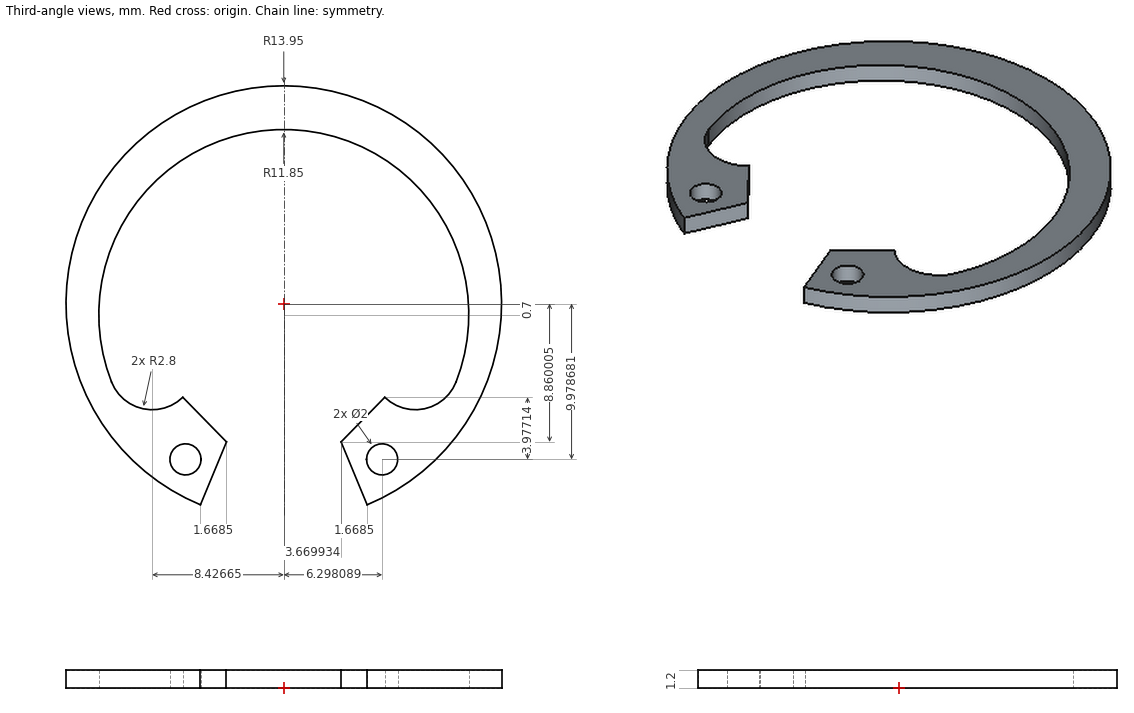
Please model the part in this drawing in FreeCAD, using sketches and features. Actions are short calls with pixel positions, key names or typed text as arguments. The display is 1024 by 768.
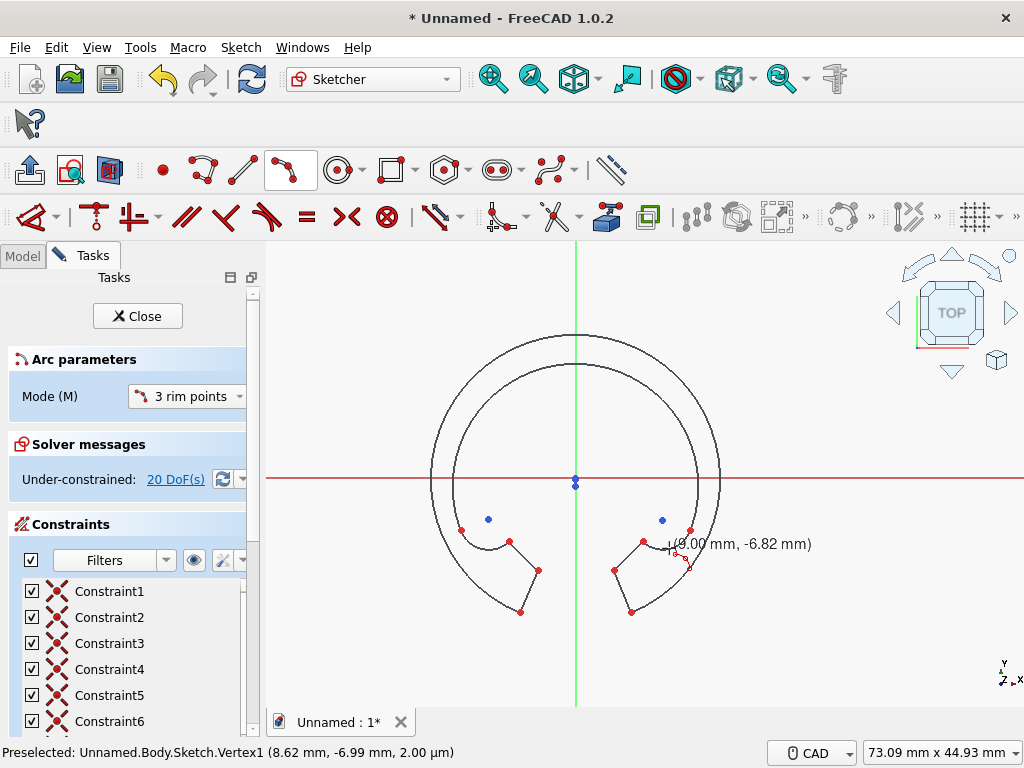
click(338, 170)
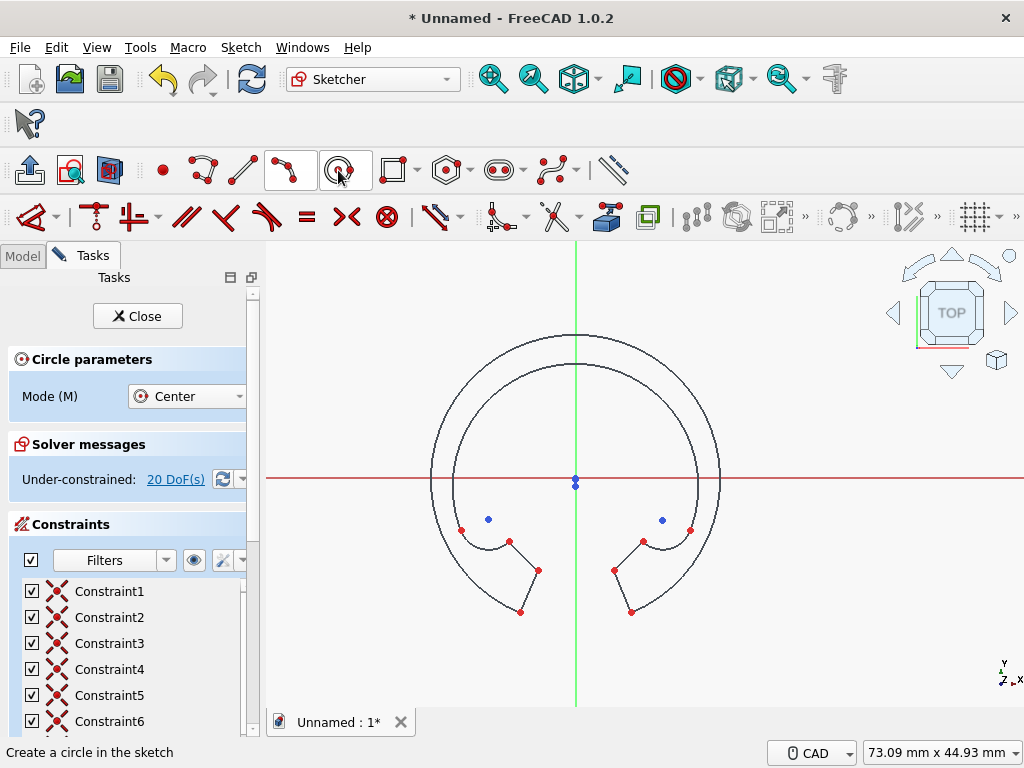
scroll(641, 582, up, 4)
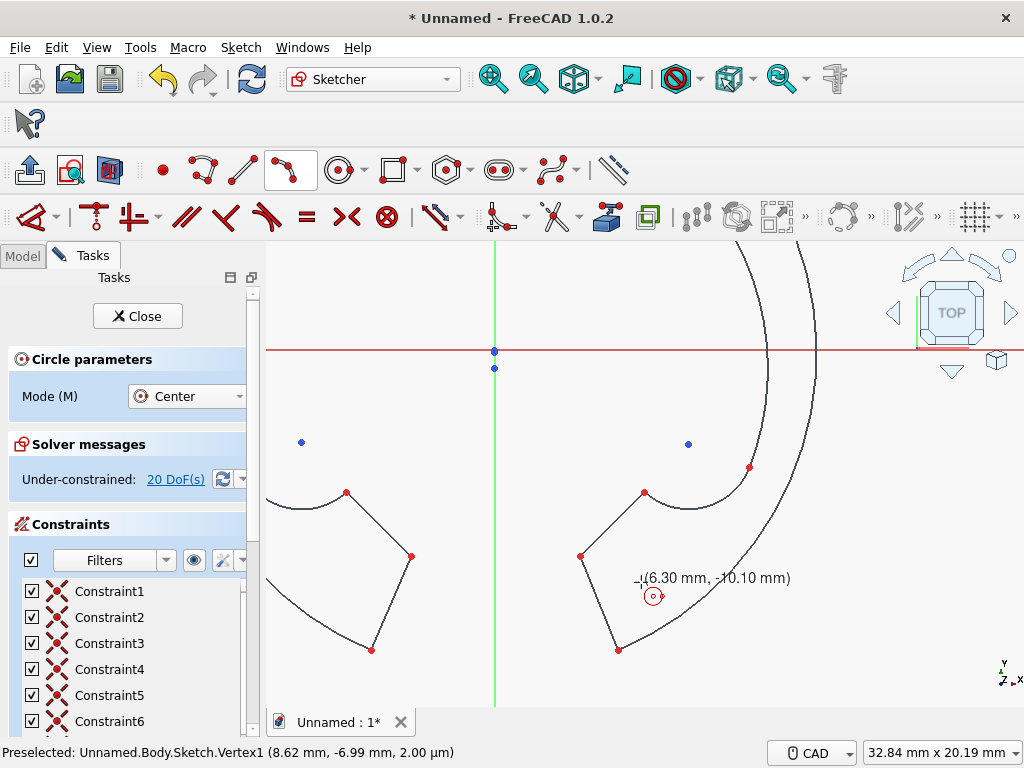
click(640, 581)
click(657, 564)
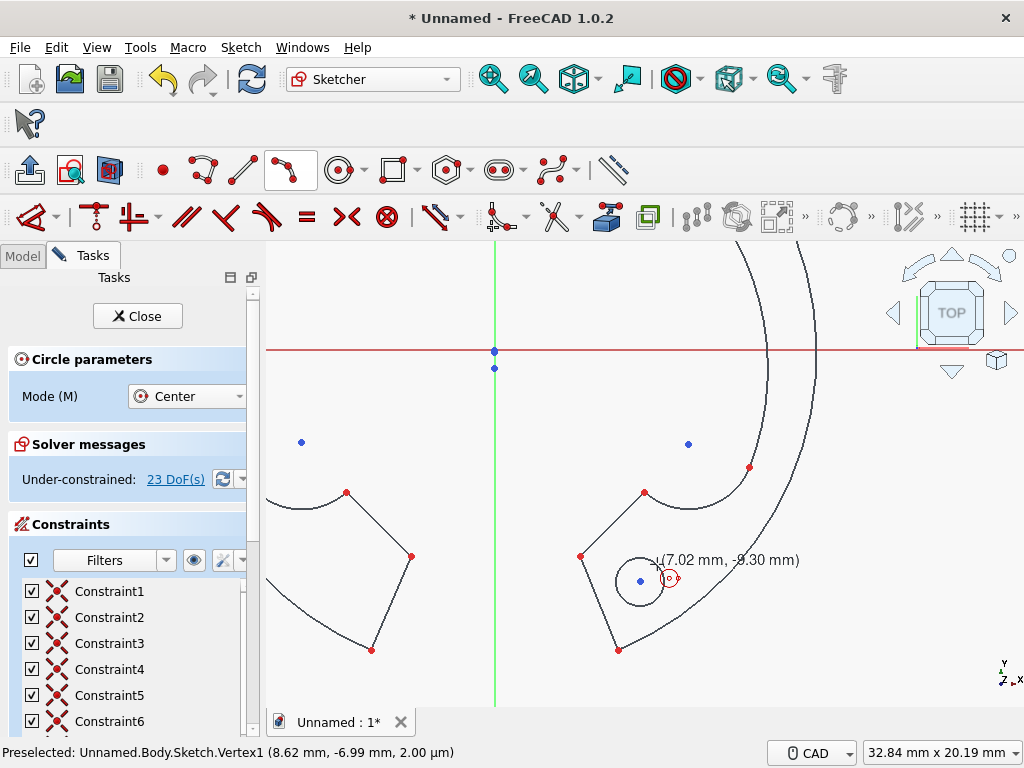
click(350, 581)
click(366, 564)
key(Escape)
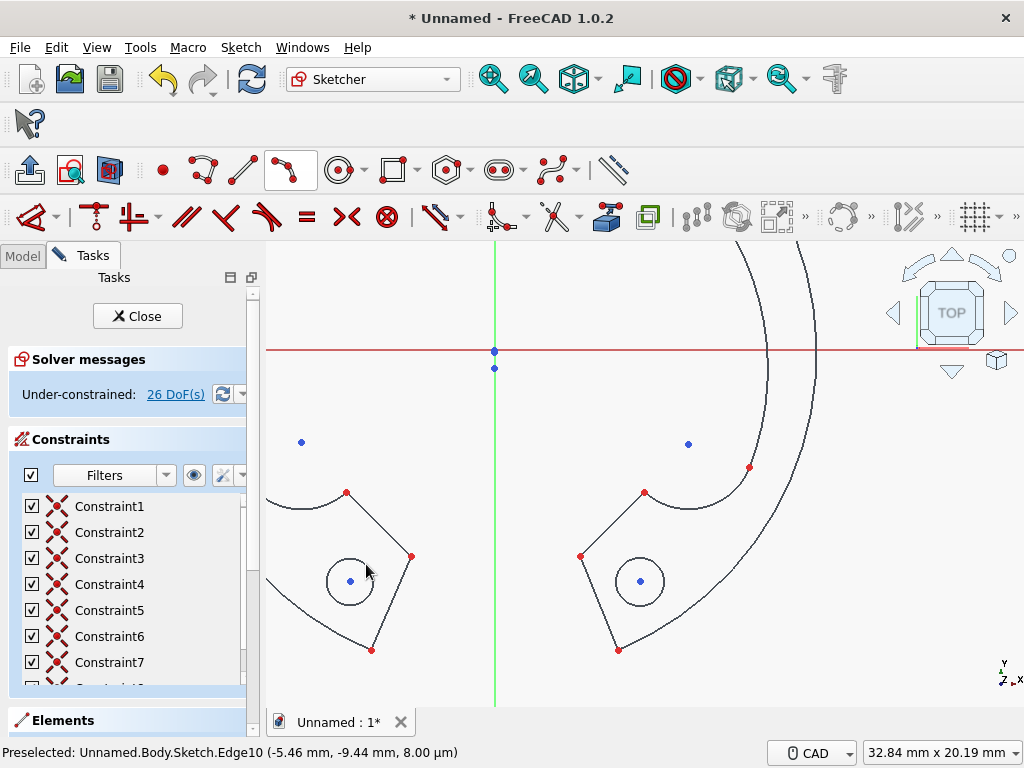
click(312, 509)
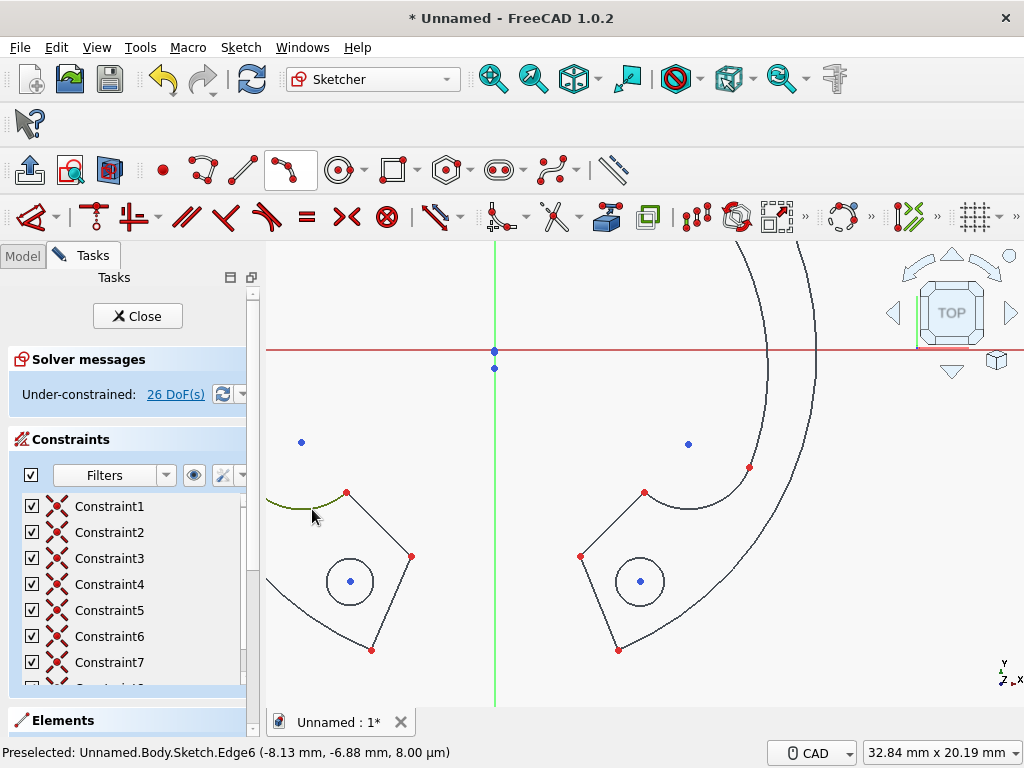
scroll(643, 585, down, 4)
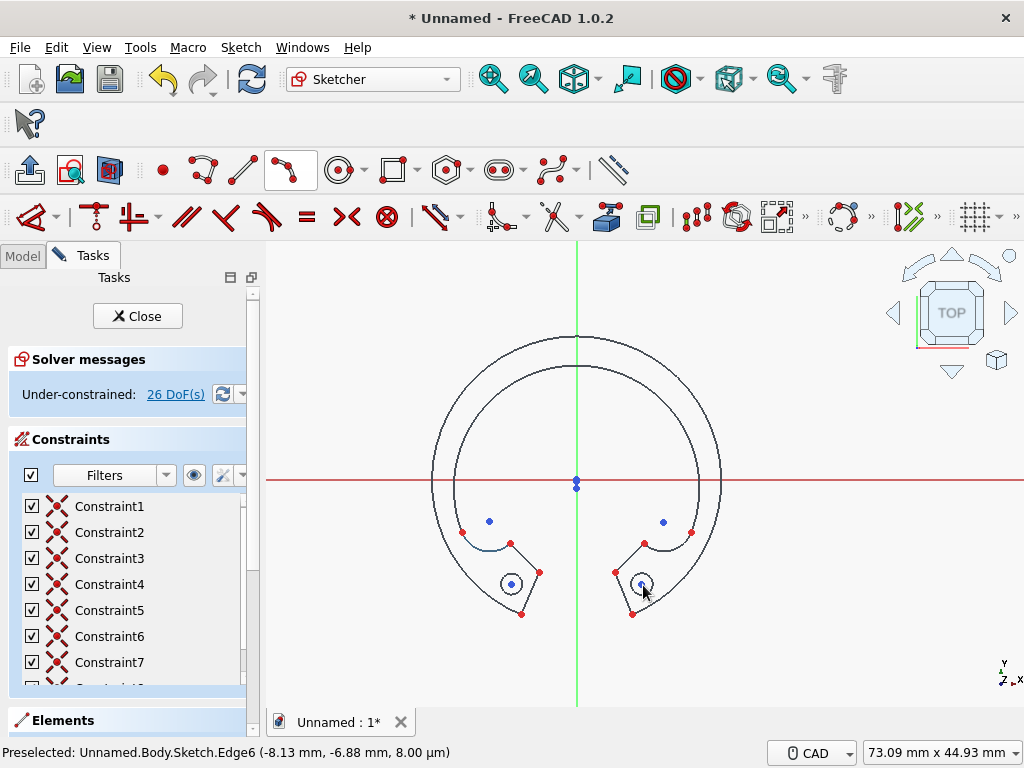
click(663, 401)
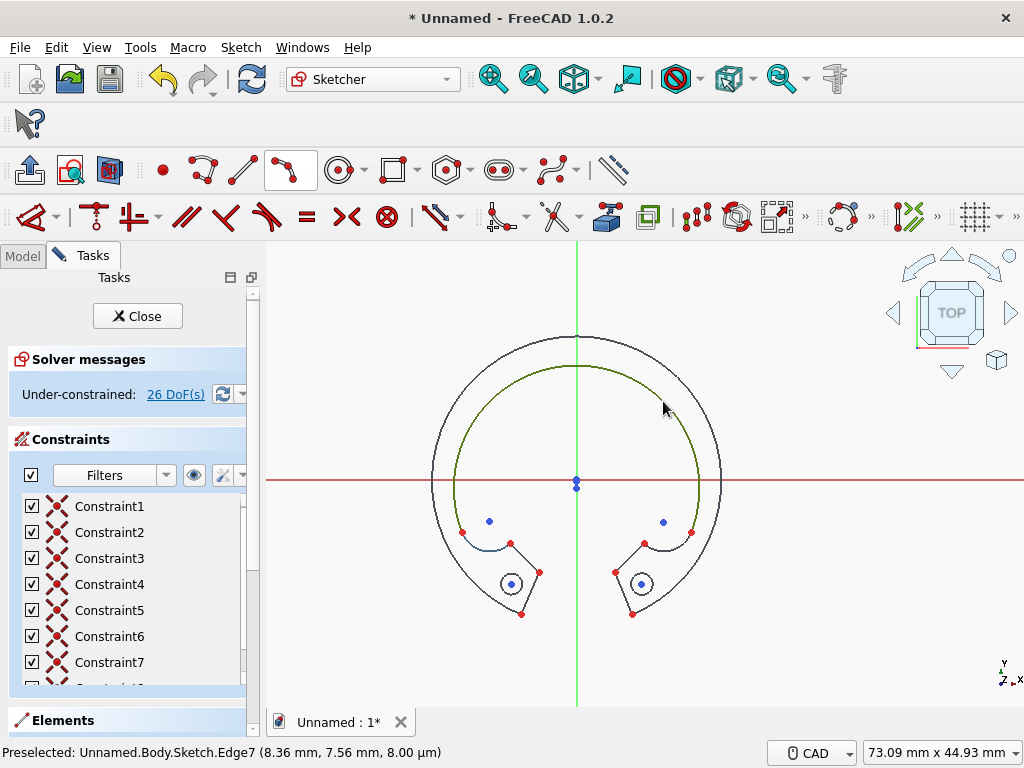
click(268, 218)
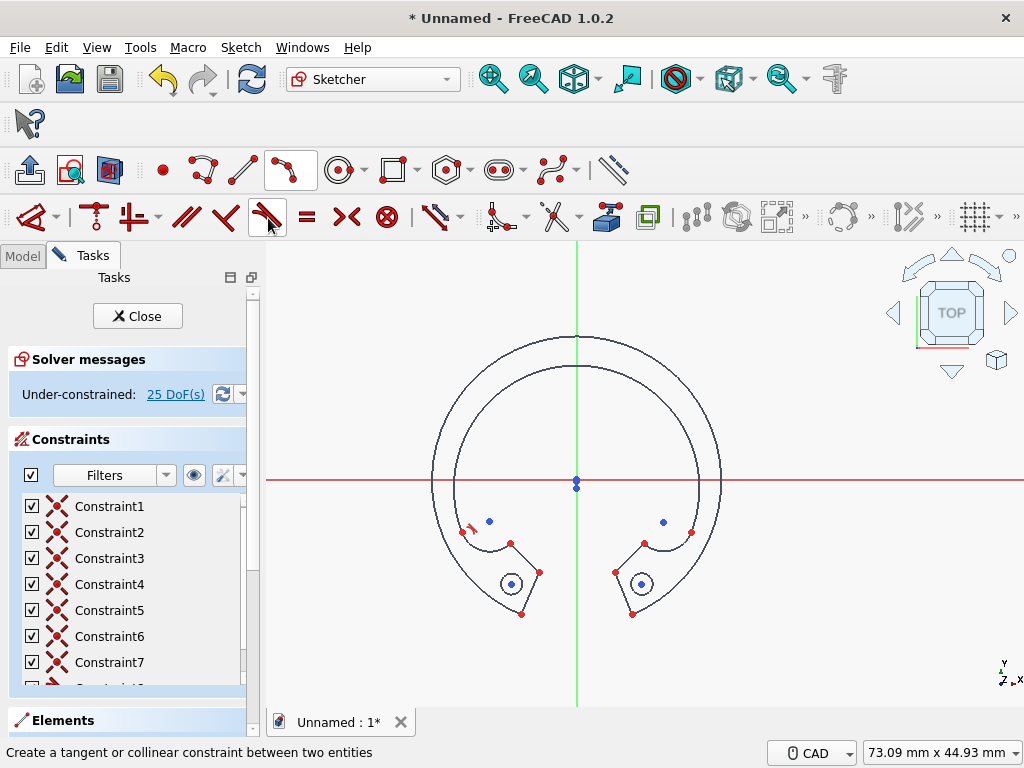
click(663, 401)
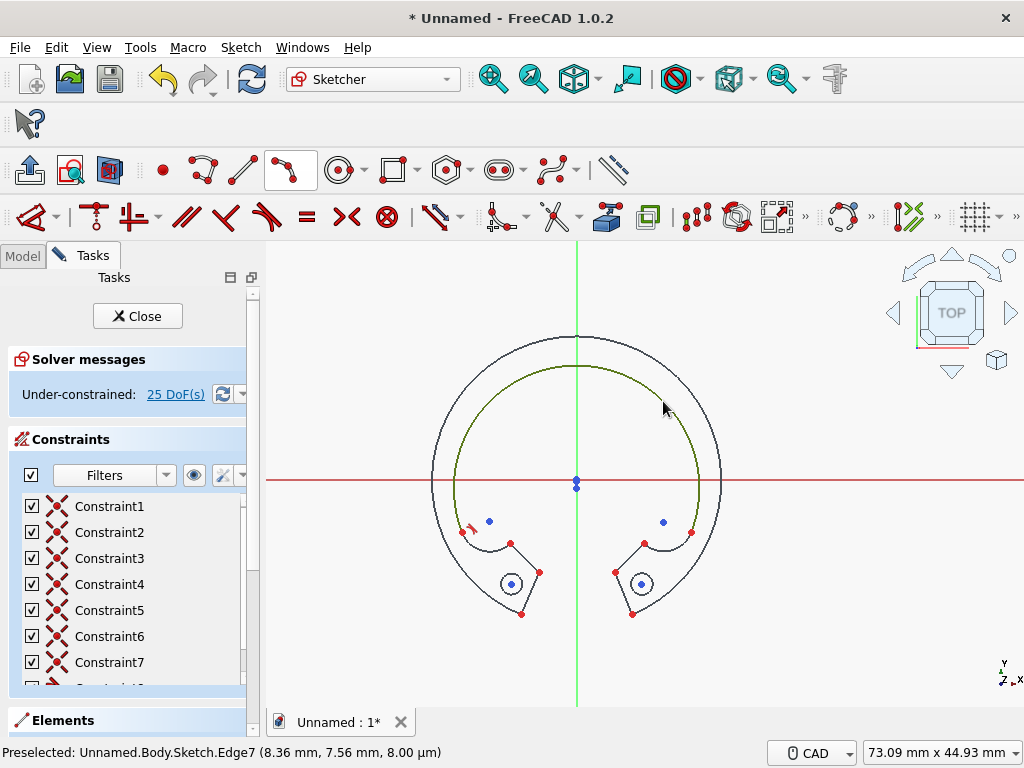
click(659, 551)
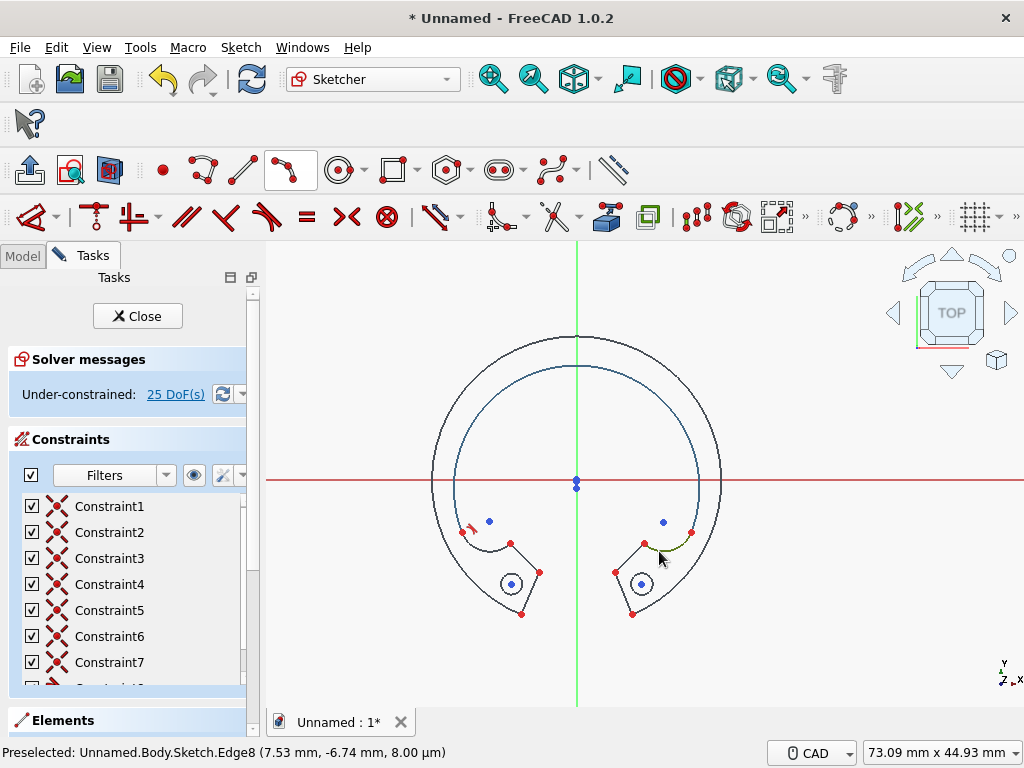
key(t)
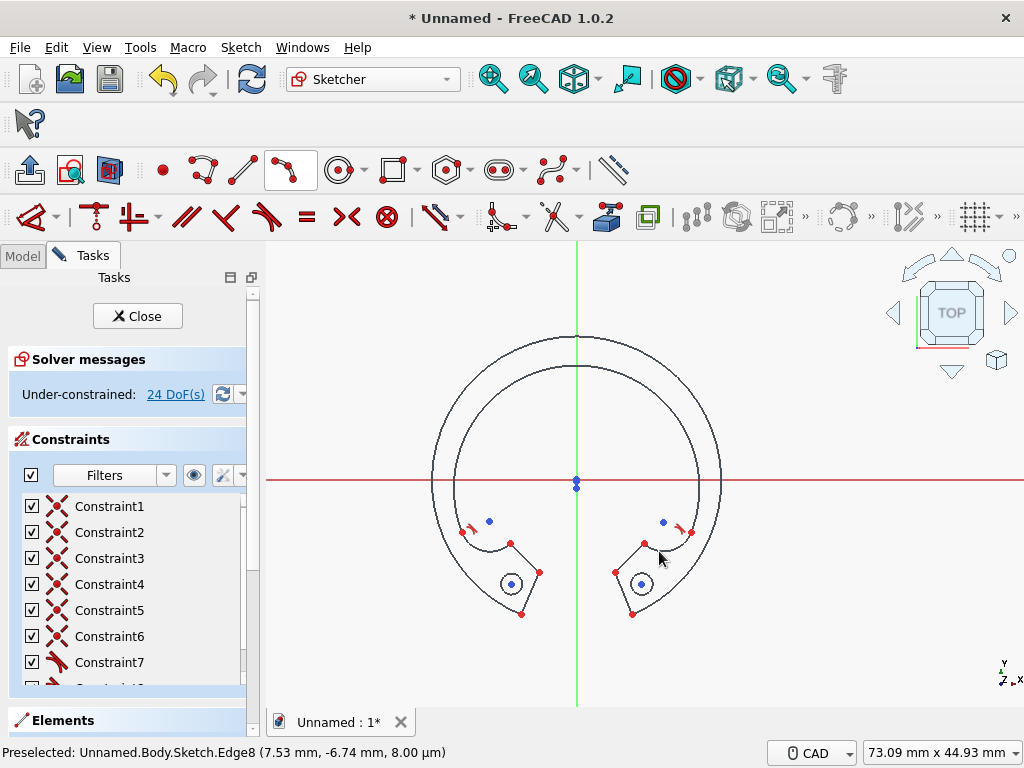
scroll(577, 481, up, 7)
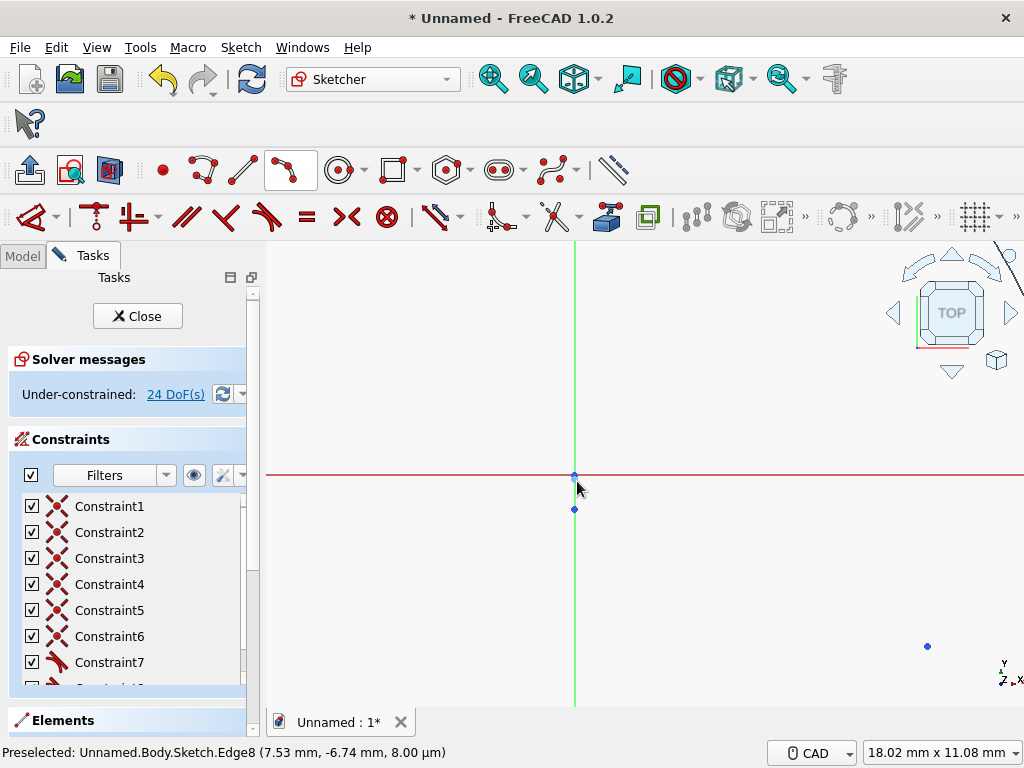
drag(564, 465, 585, 490)